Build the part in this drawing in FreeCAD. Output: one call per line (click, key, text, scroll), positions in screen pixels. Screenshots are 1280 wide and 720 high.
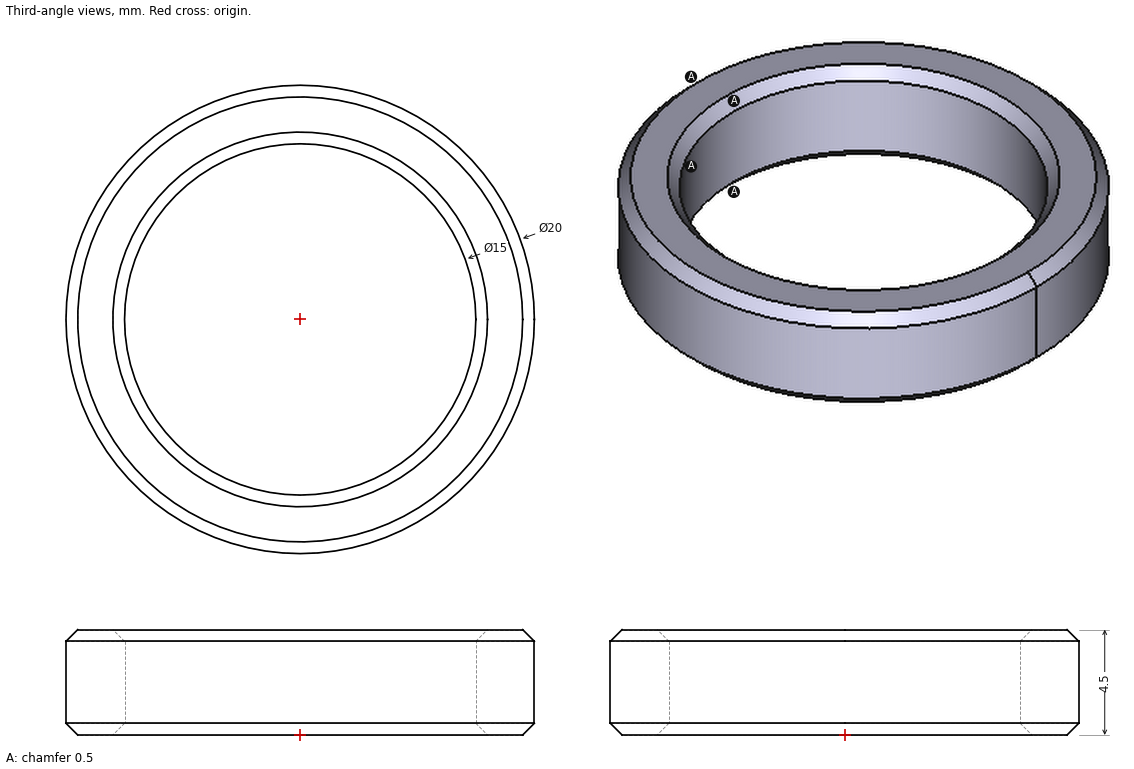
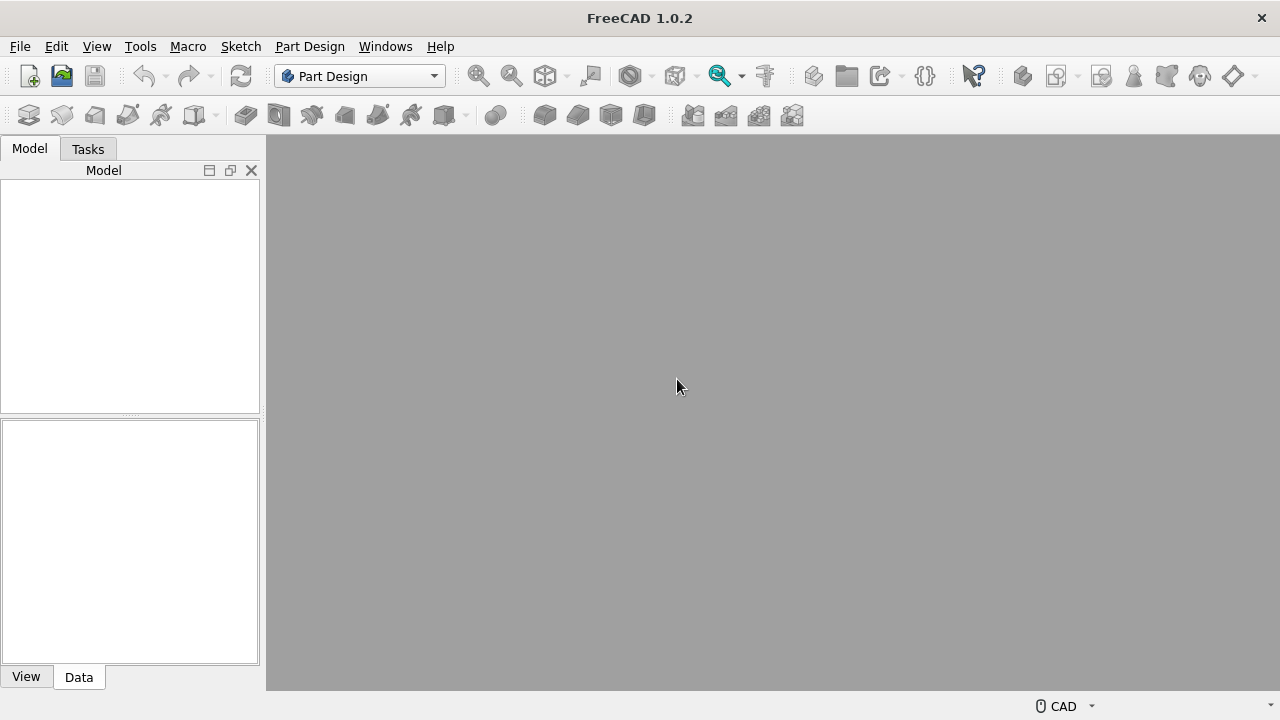
click(29, 76)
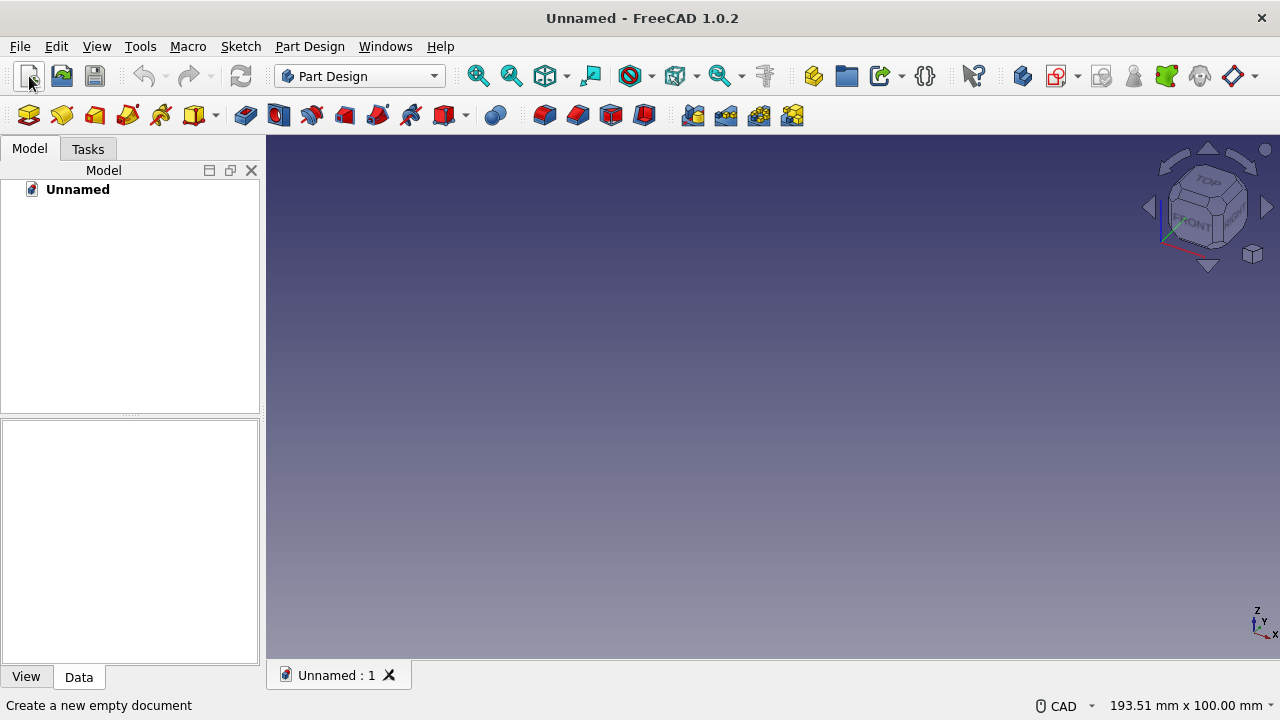
click(1056, 76)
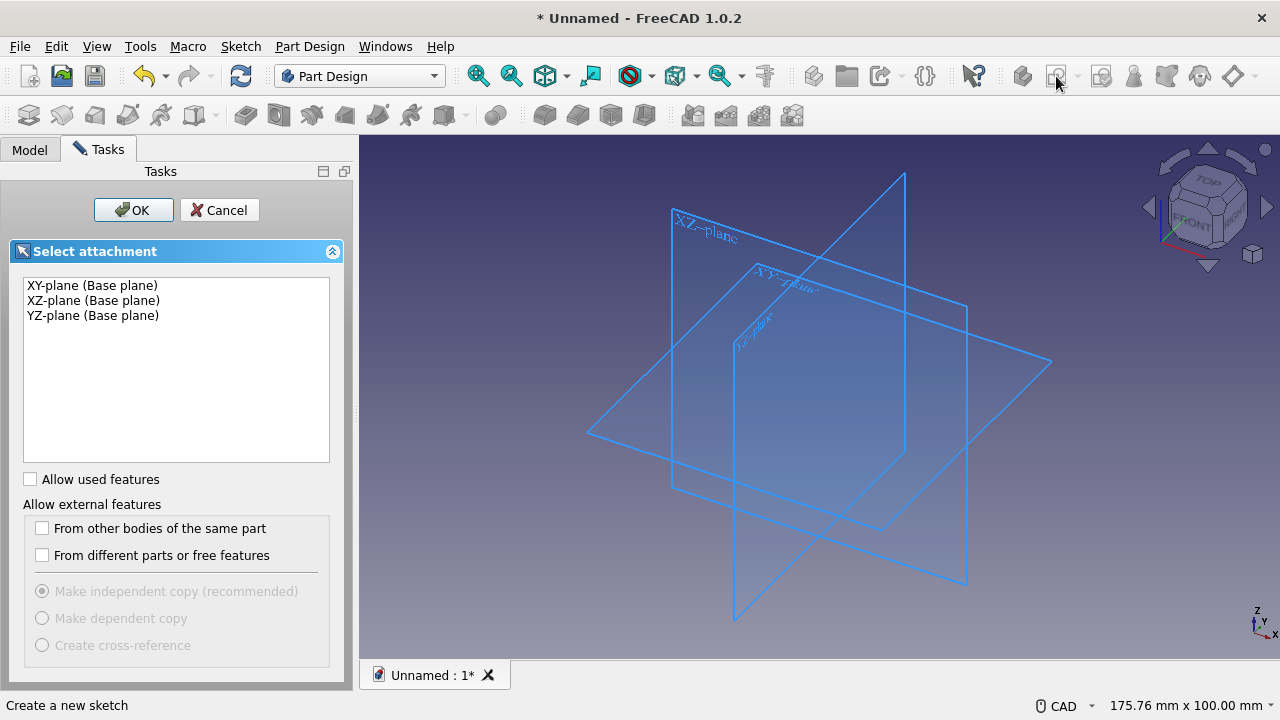
click(84, 286)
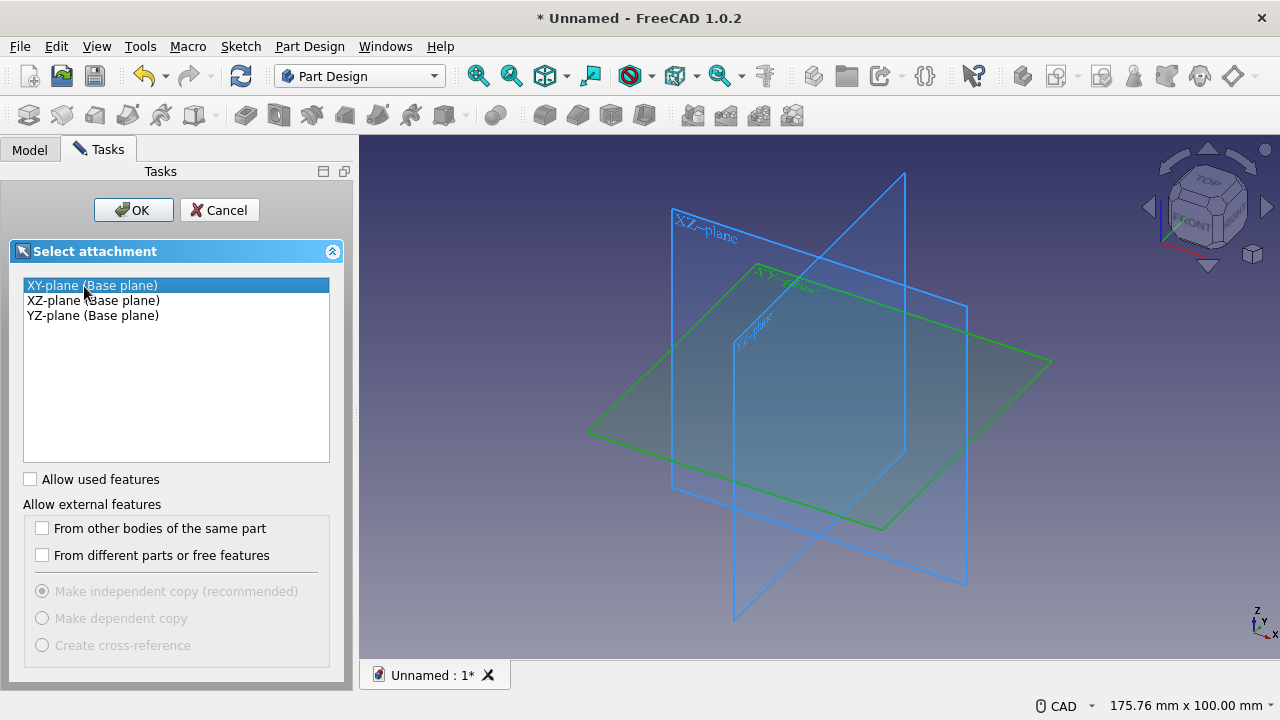
click(134, 210)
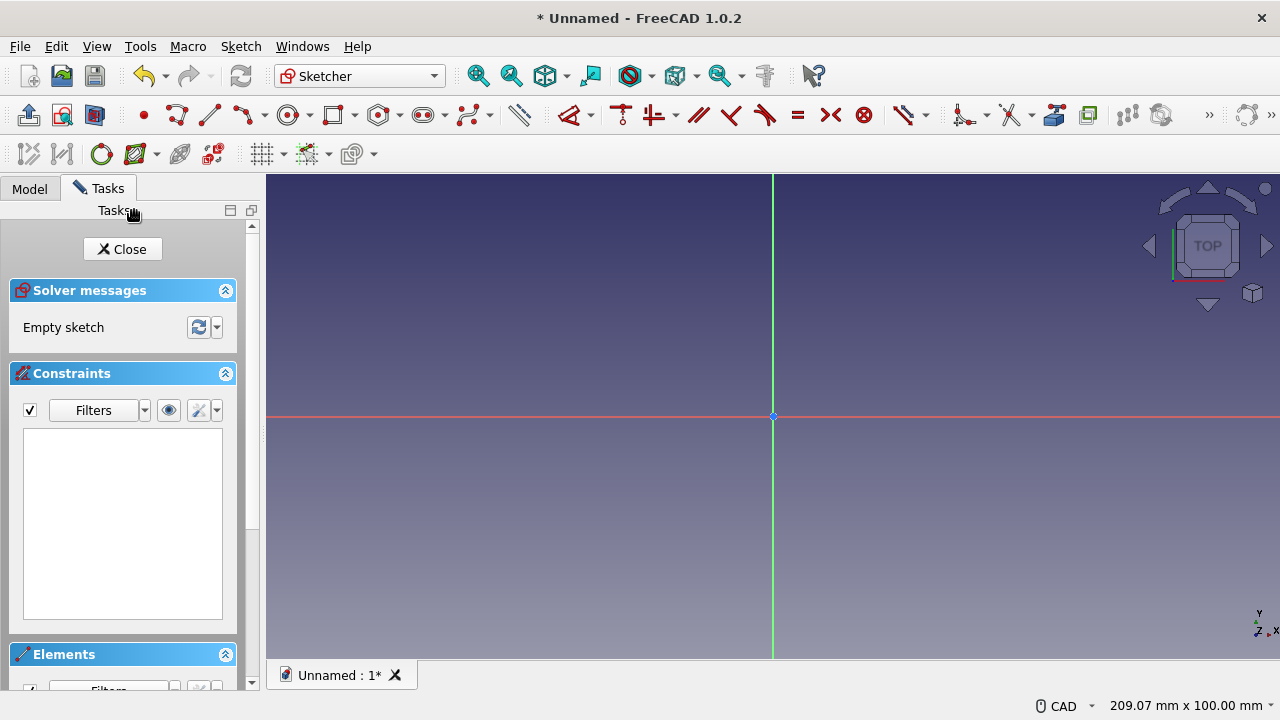
scroll(803, 416, up, 6)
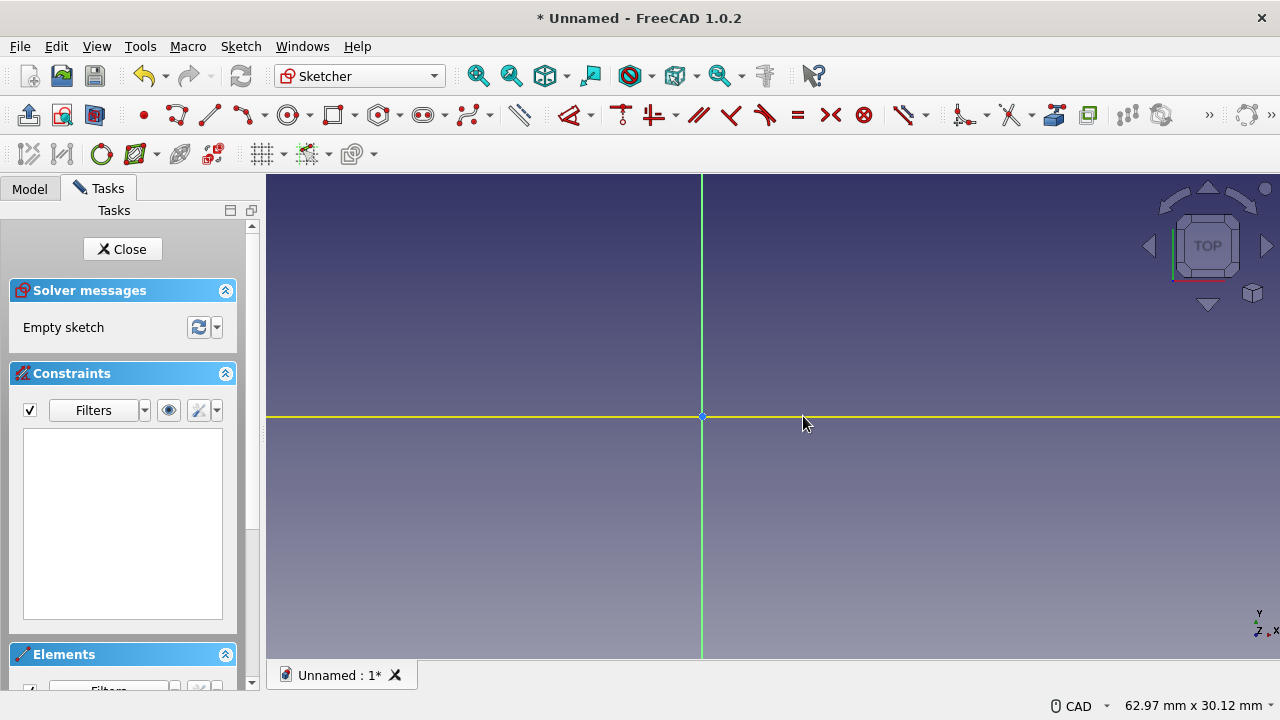
click(288, 116)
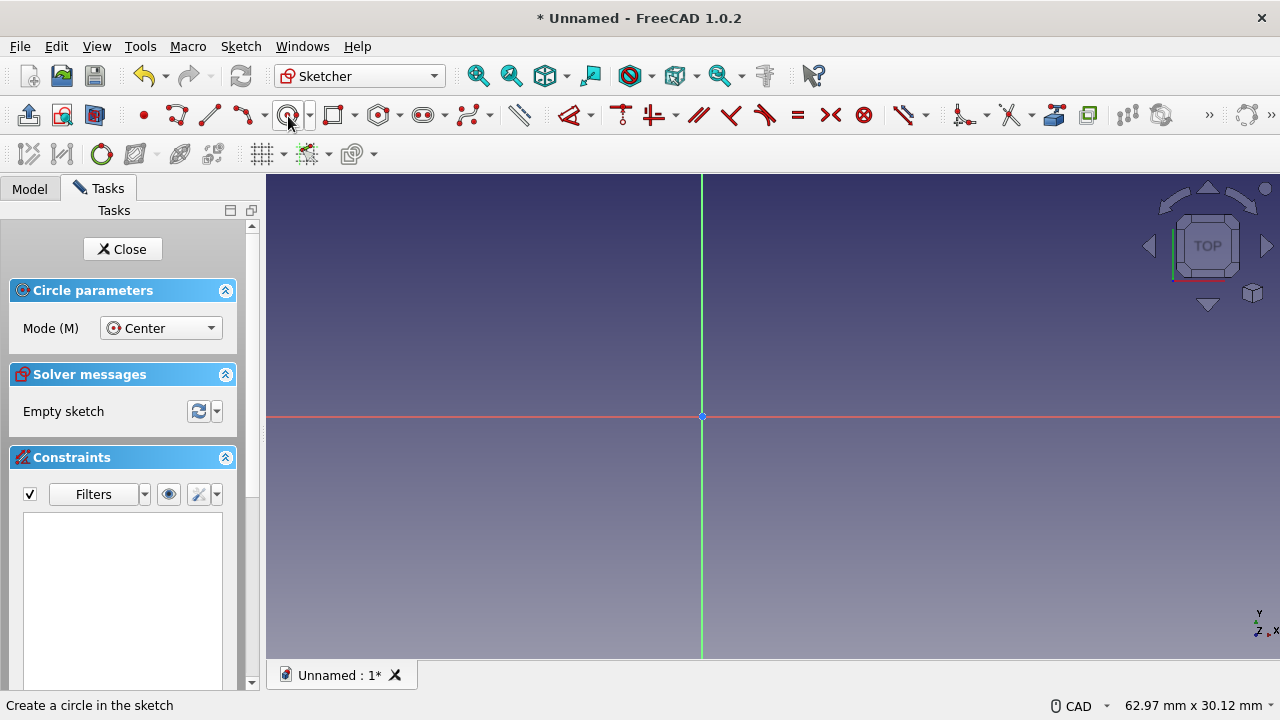
click(702, 416)
move(816, 303)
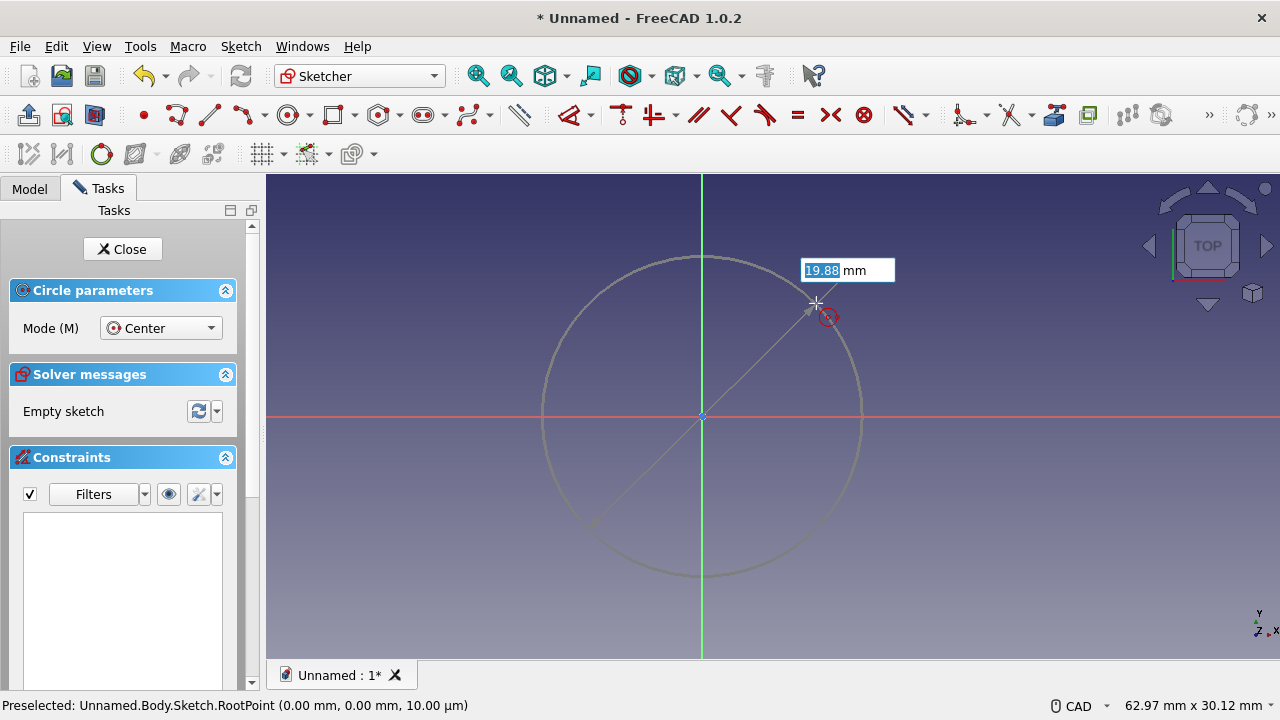
text(20)
key(Return)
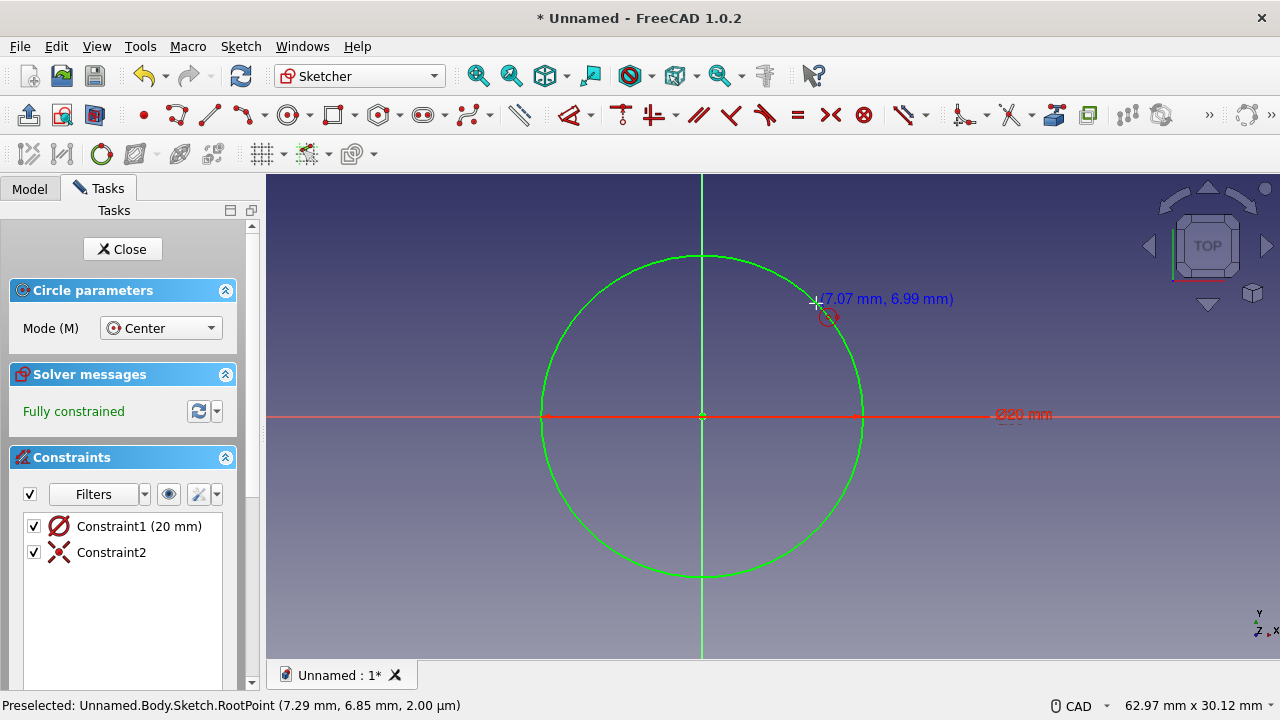
click(702, 416)
move(788, 331)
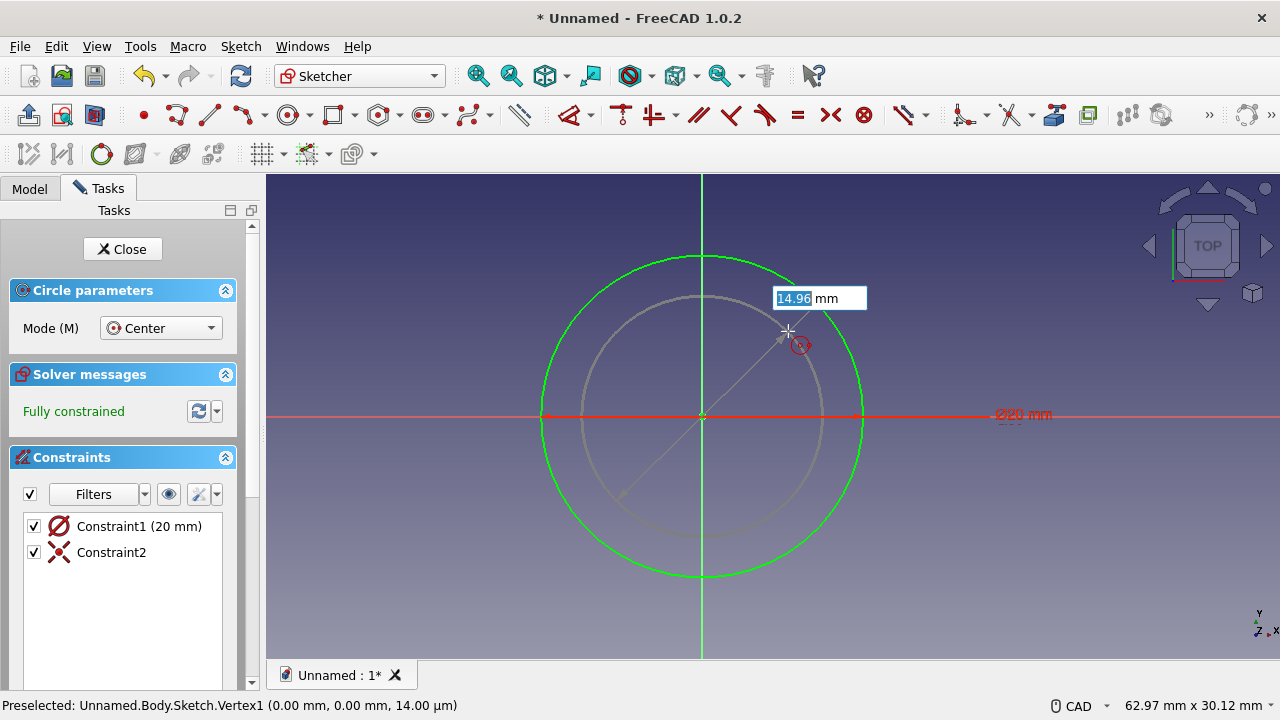
text(15)
key(Return)
key(Escape)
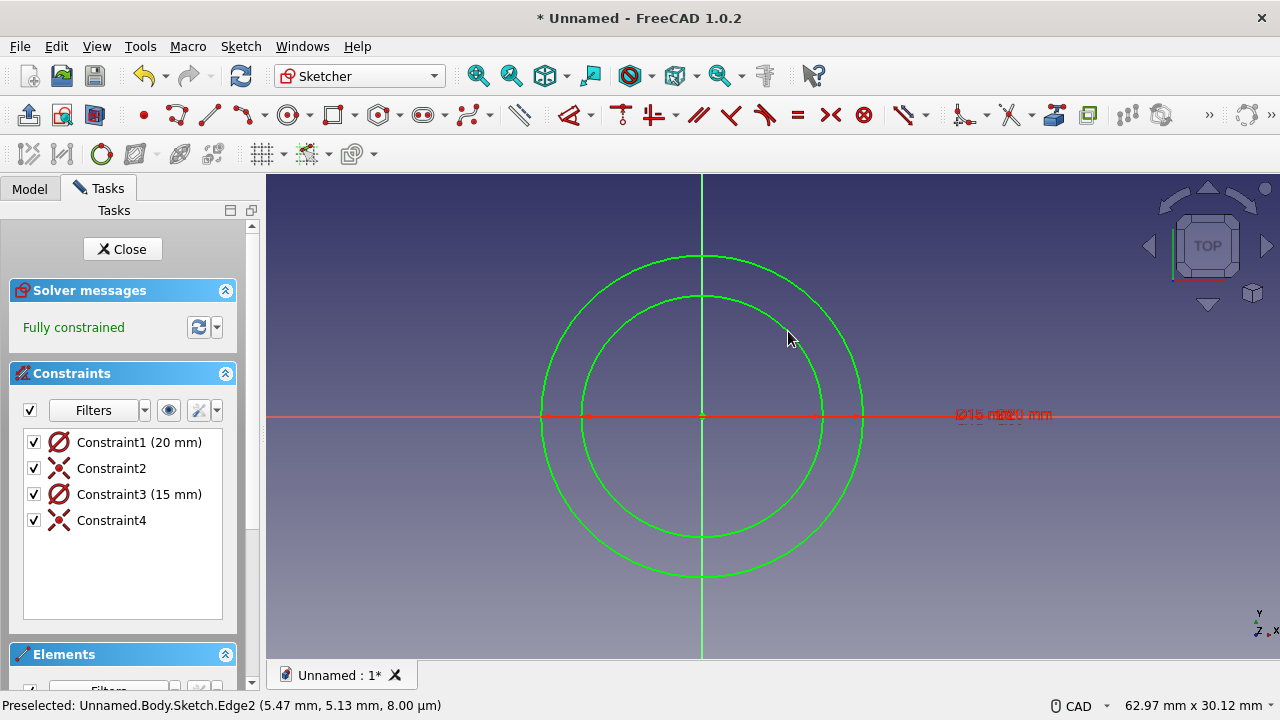
click(123, 249)